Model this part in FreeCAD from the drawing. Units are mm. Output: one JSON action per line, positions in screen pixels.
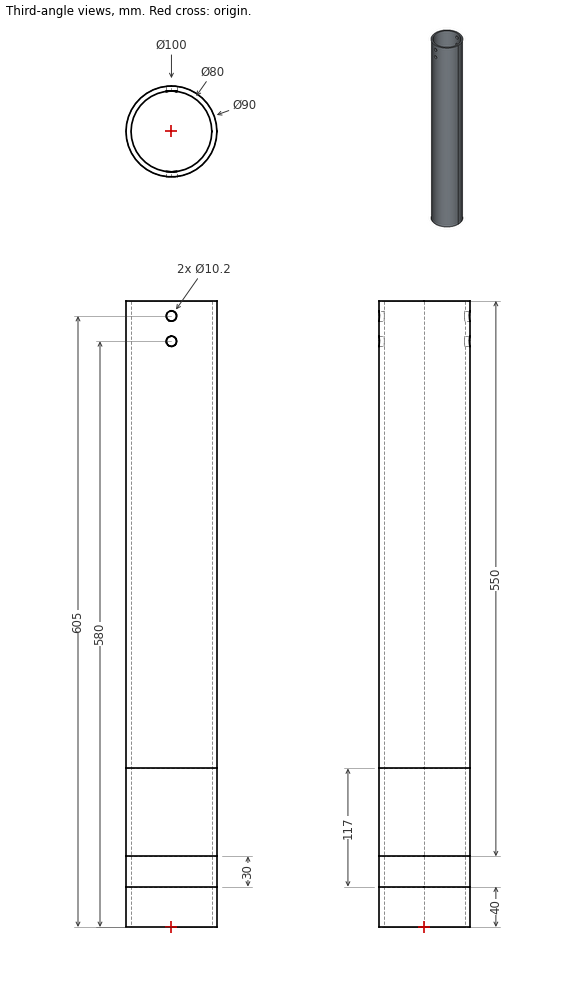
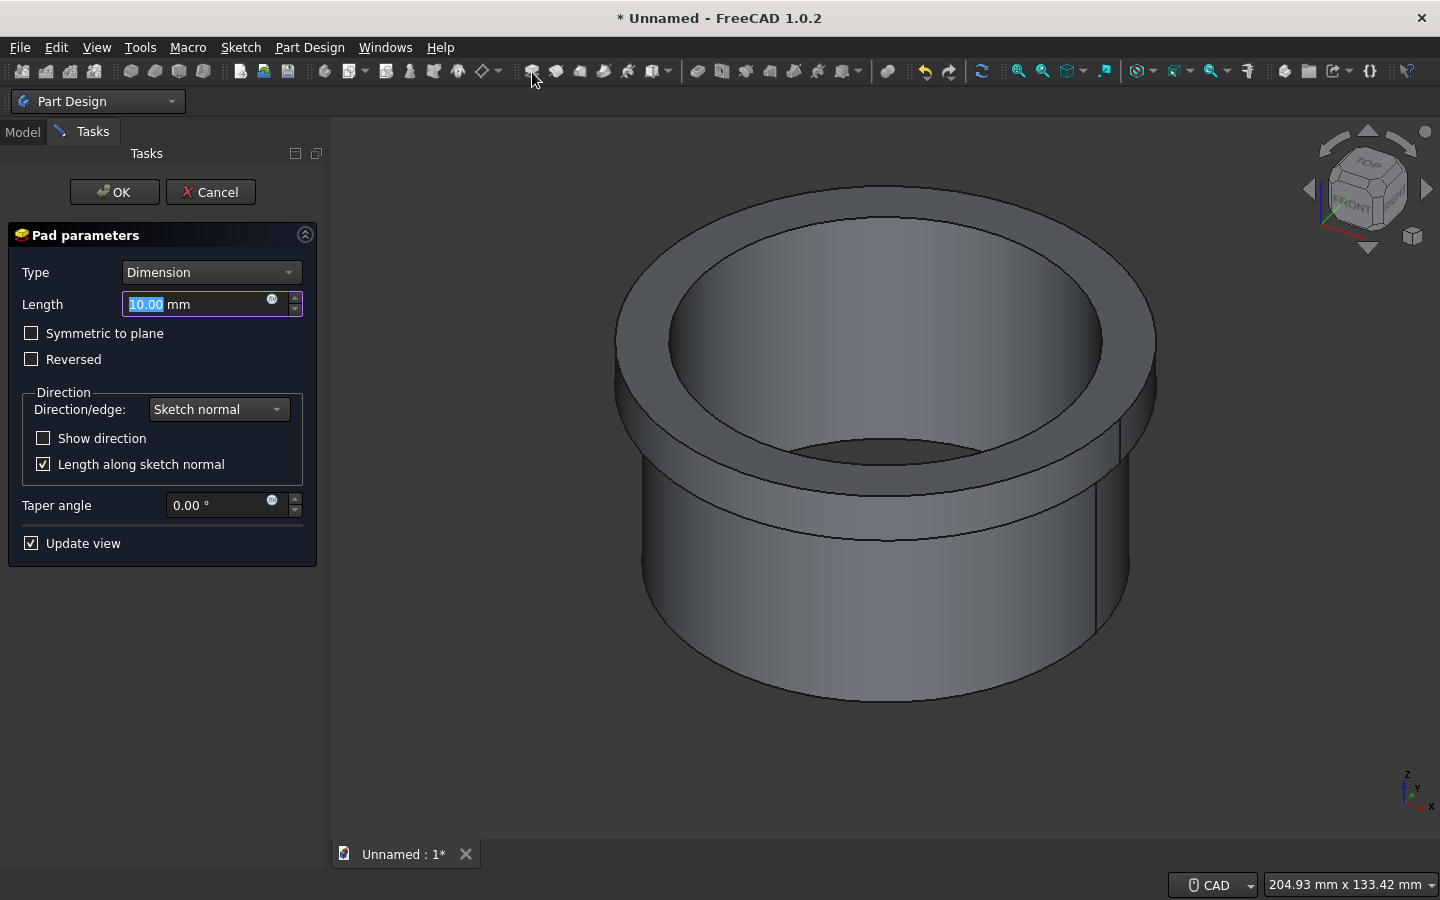
{"action": "type", "text": "30"}
{"action": "key", "text": "Tab"}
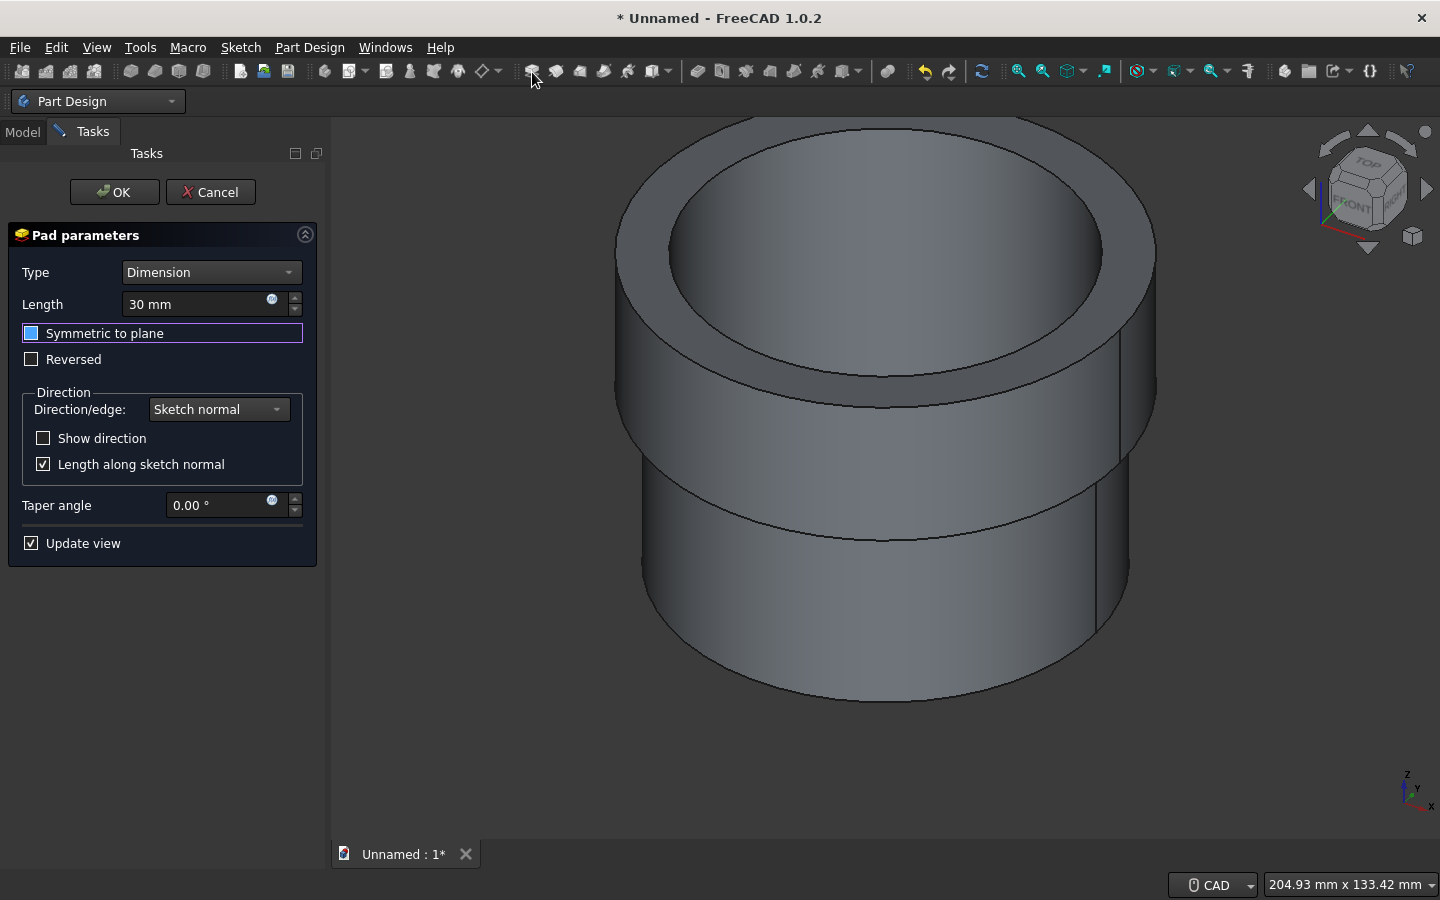
{"action": "left_click", "coordinate": [115, 192]}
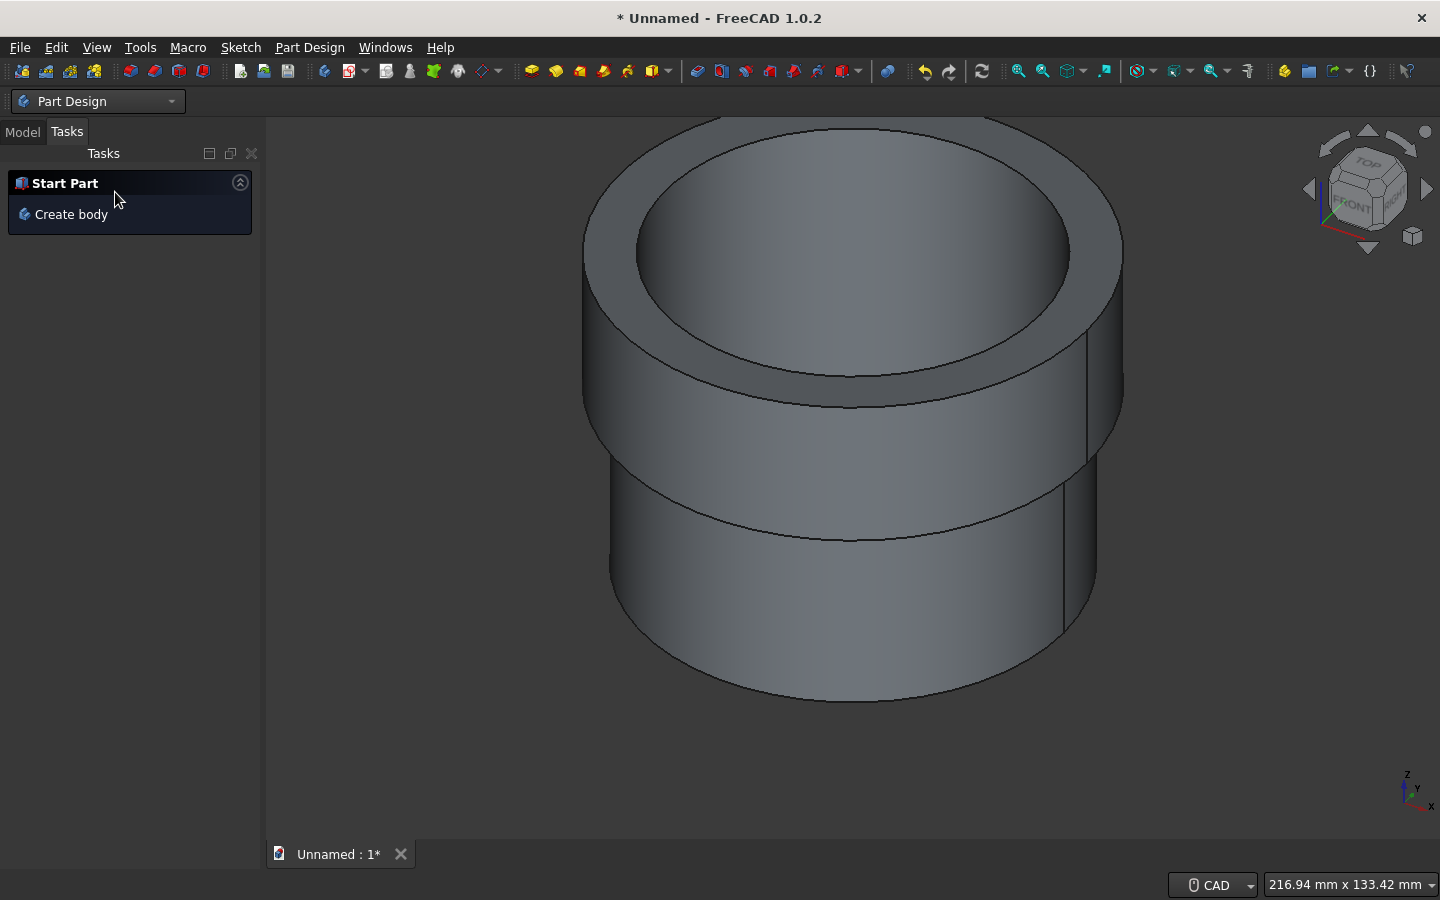
{"action": "key", "text": "v f"}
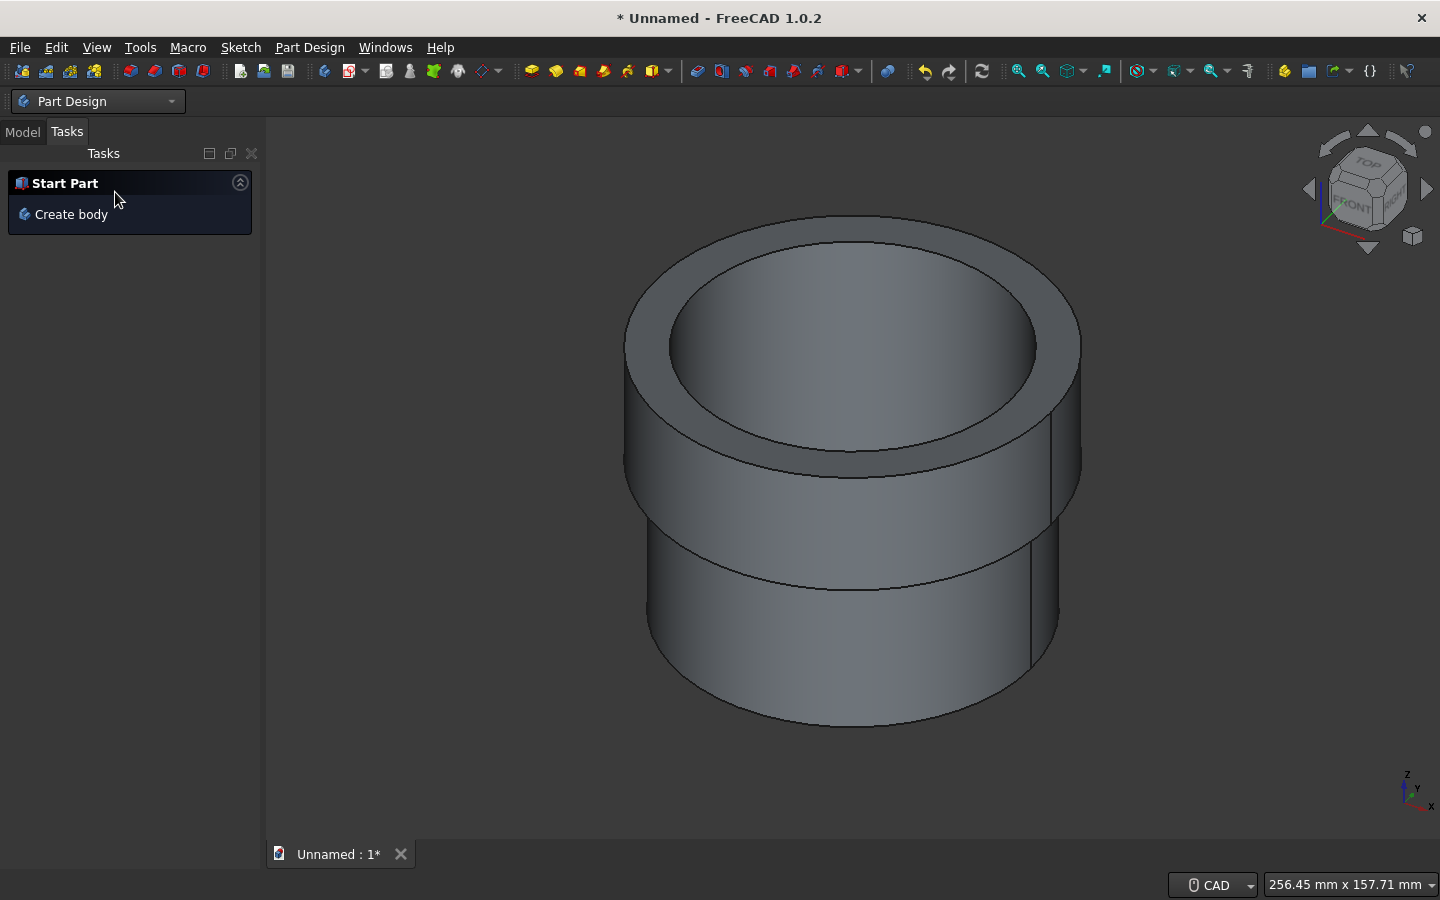
{"action": "left_click", "coordinate": [650, 322]}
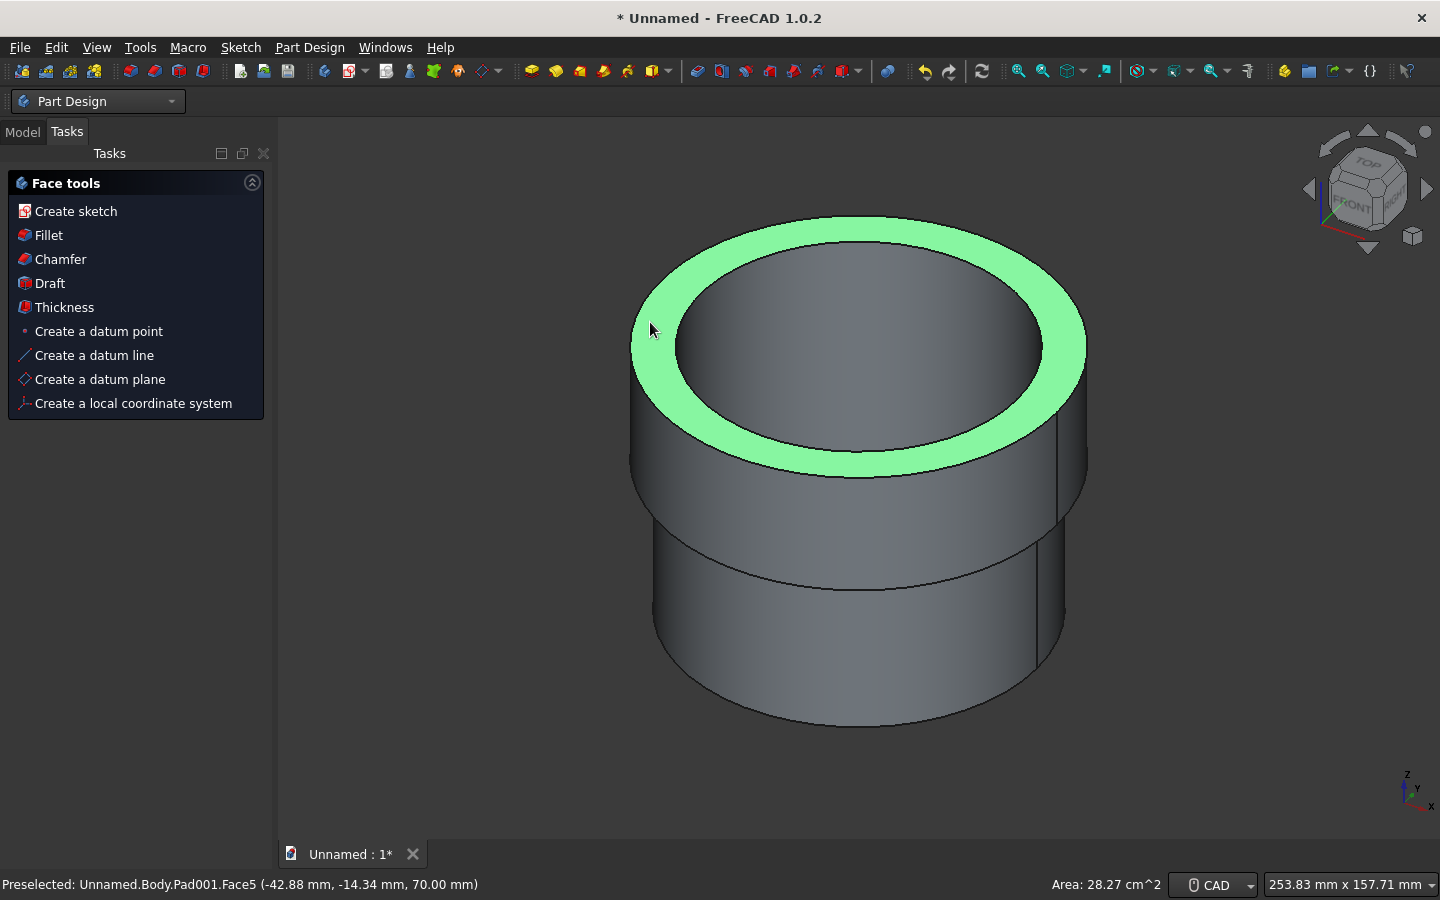
{"action": "left_click", "coordinate": [350, 72]}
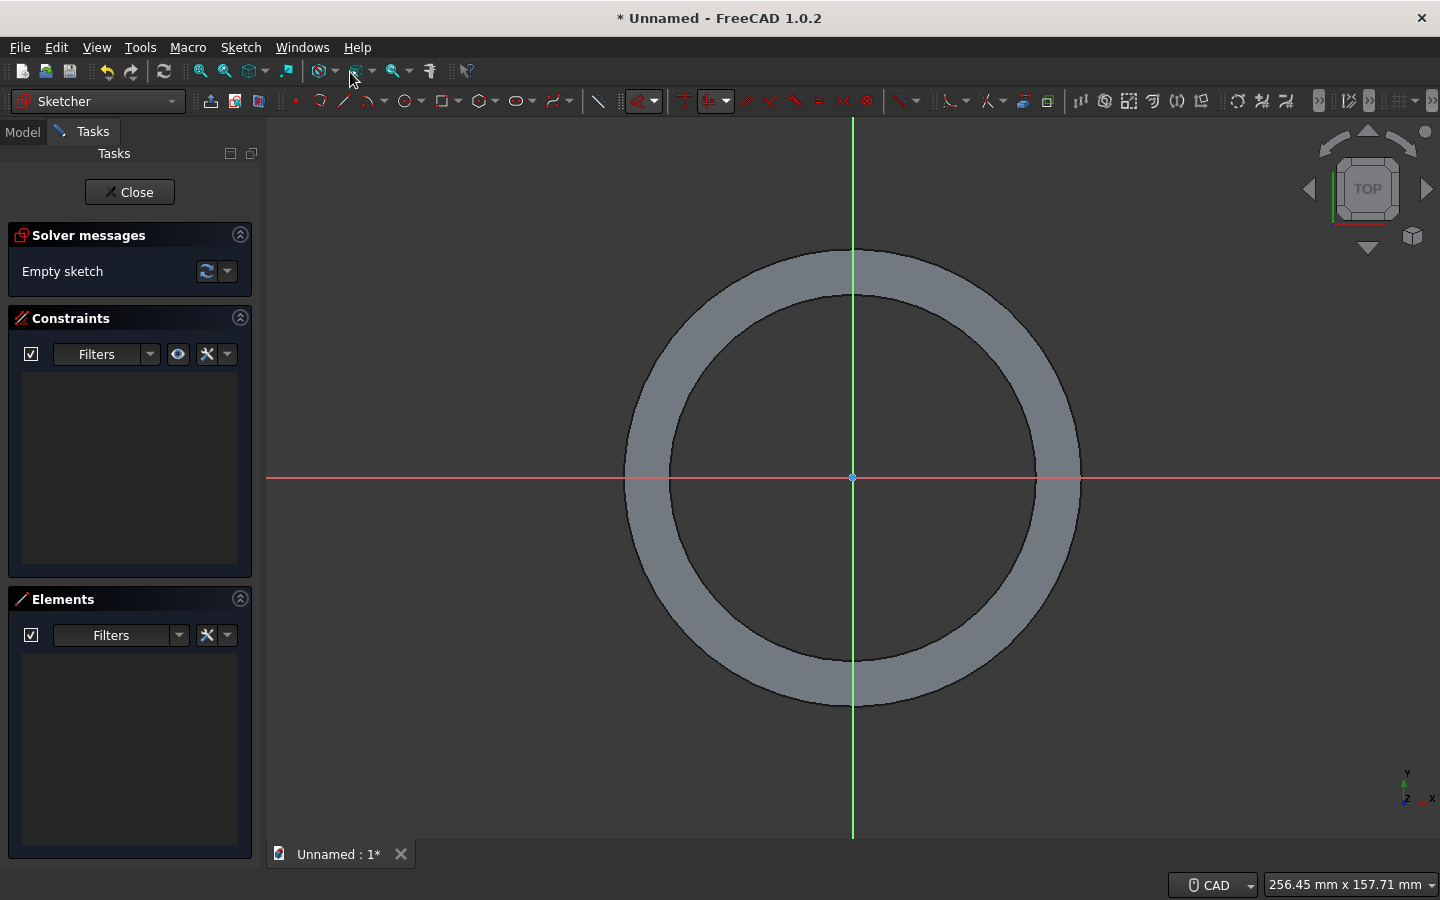
{"action": "key", "text": "g c"}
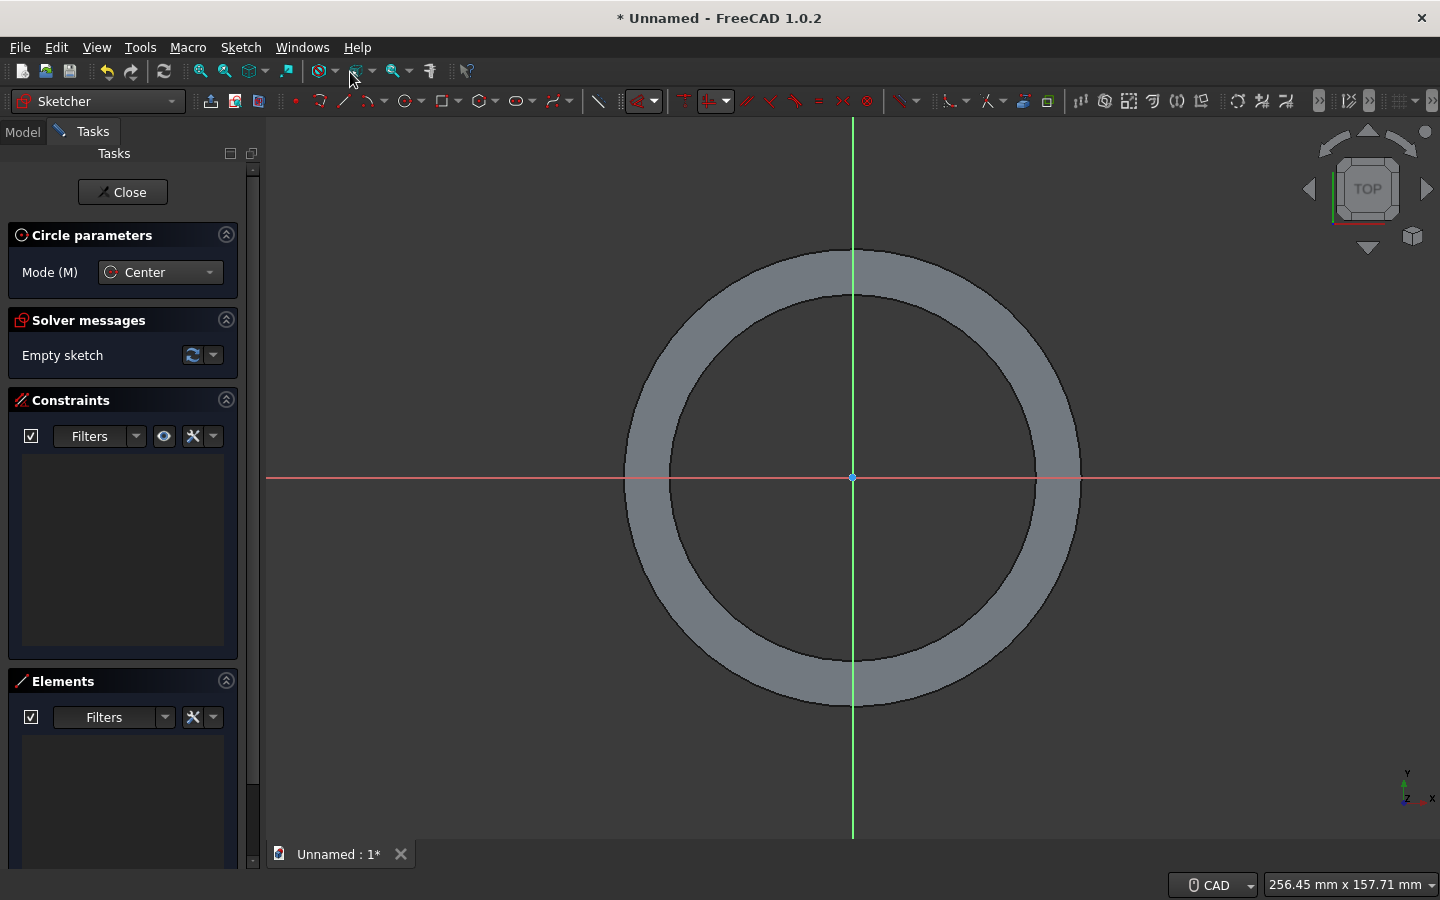
{"action": "left_click", "coordinate": [853, 478]}
{"action": "mouse_move", "coordinate": [998, 332]}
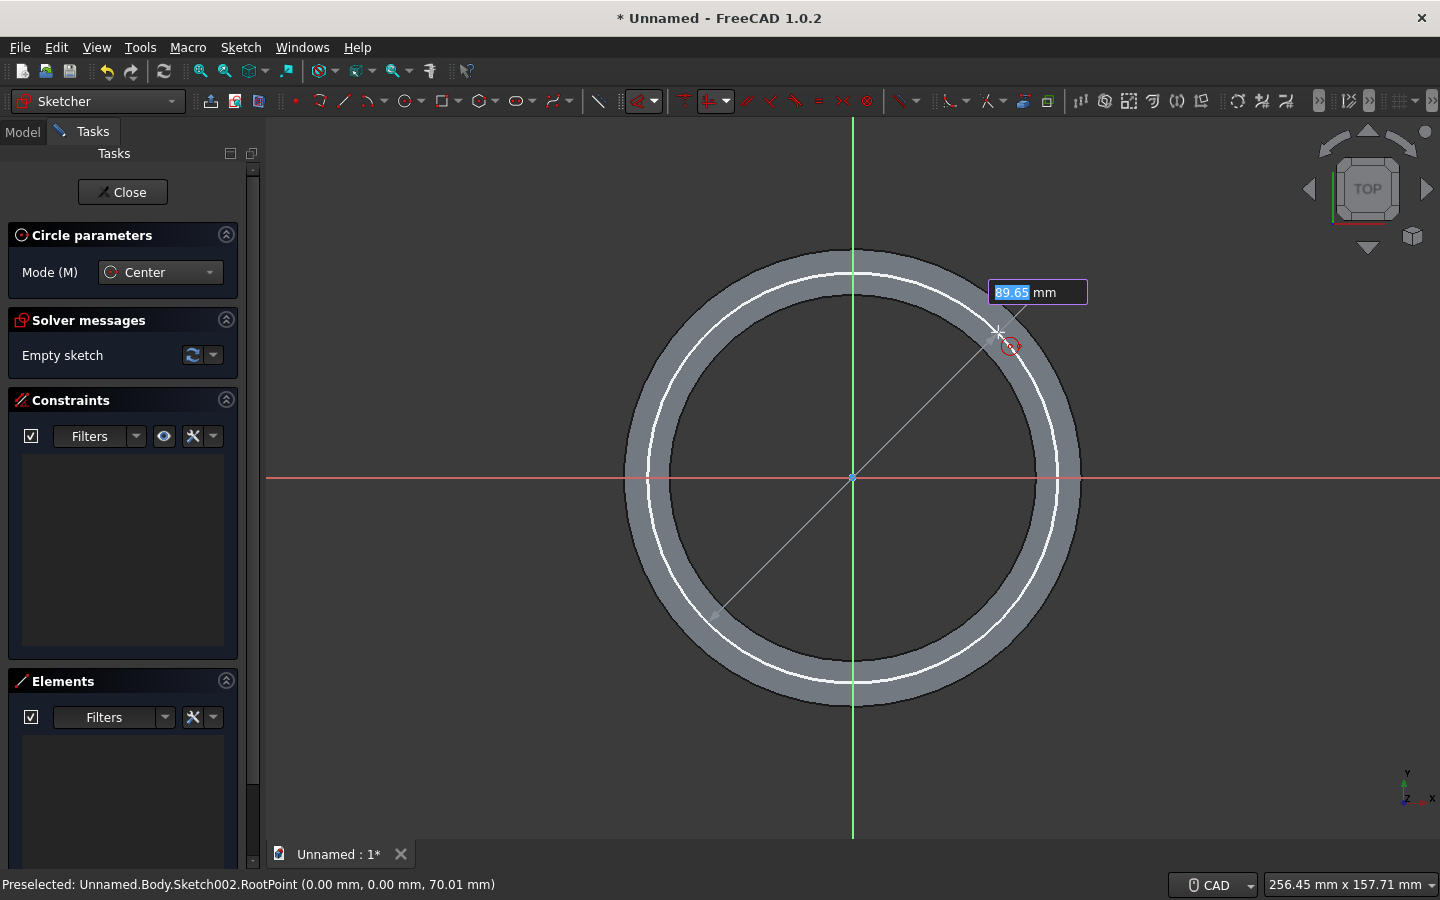
{"action": "type", "text": "90"}
{"action": "key", "text": "Return"}